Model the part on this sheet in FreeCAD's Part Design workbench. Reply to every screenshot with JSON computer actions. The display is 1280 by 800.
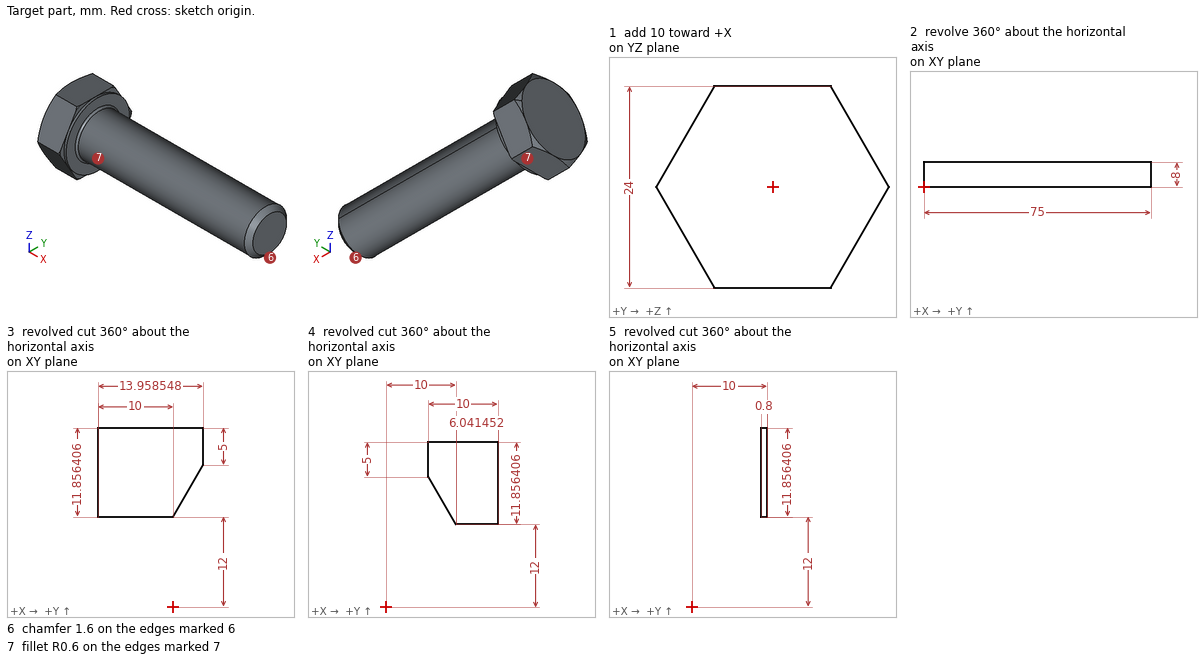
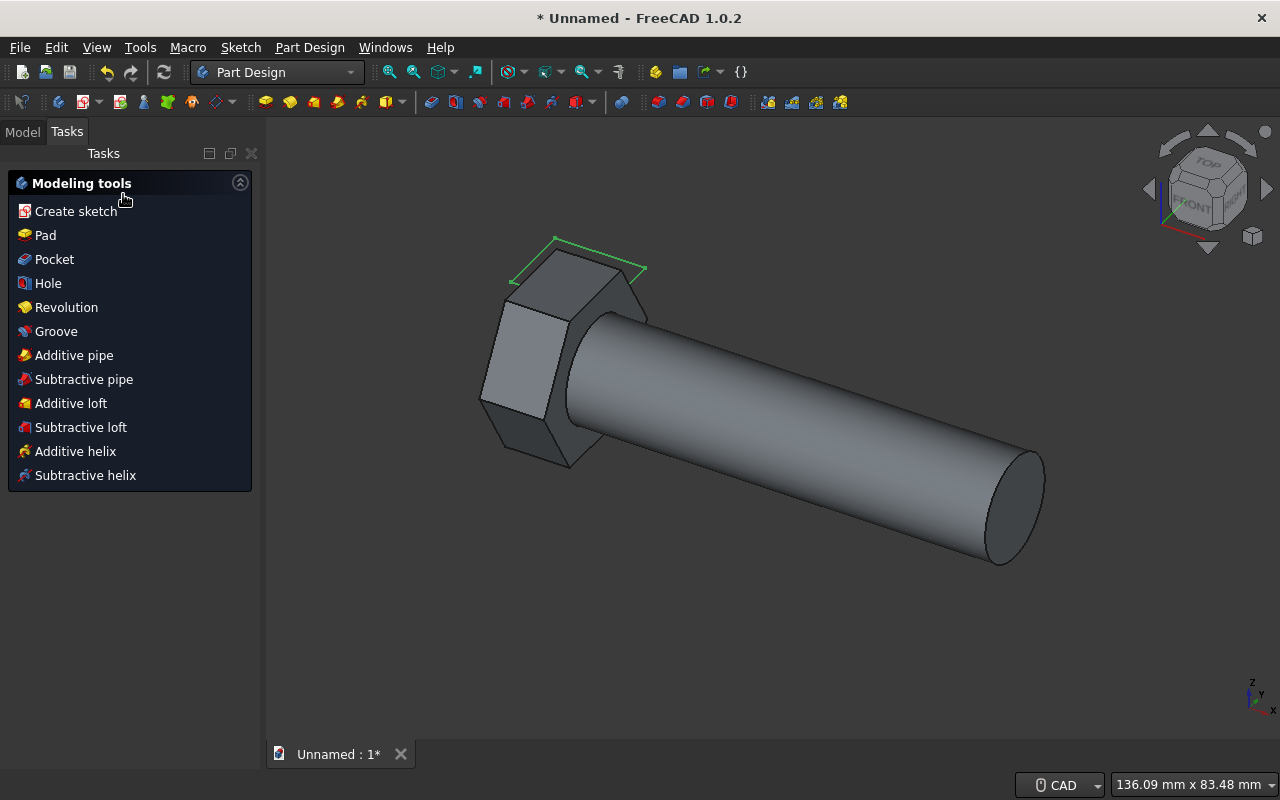
{"action": "left_click", "coordinate": [480, 102]}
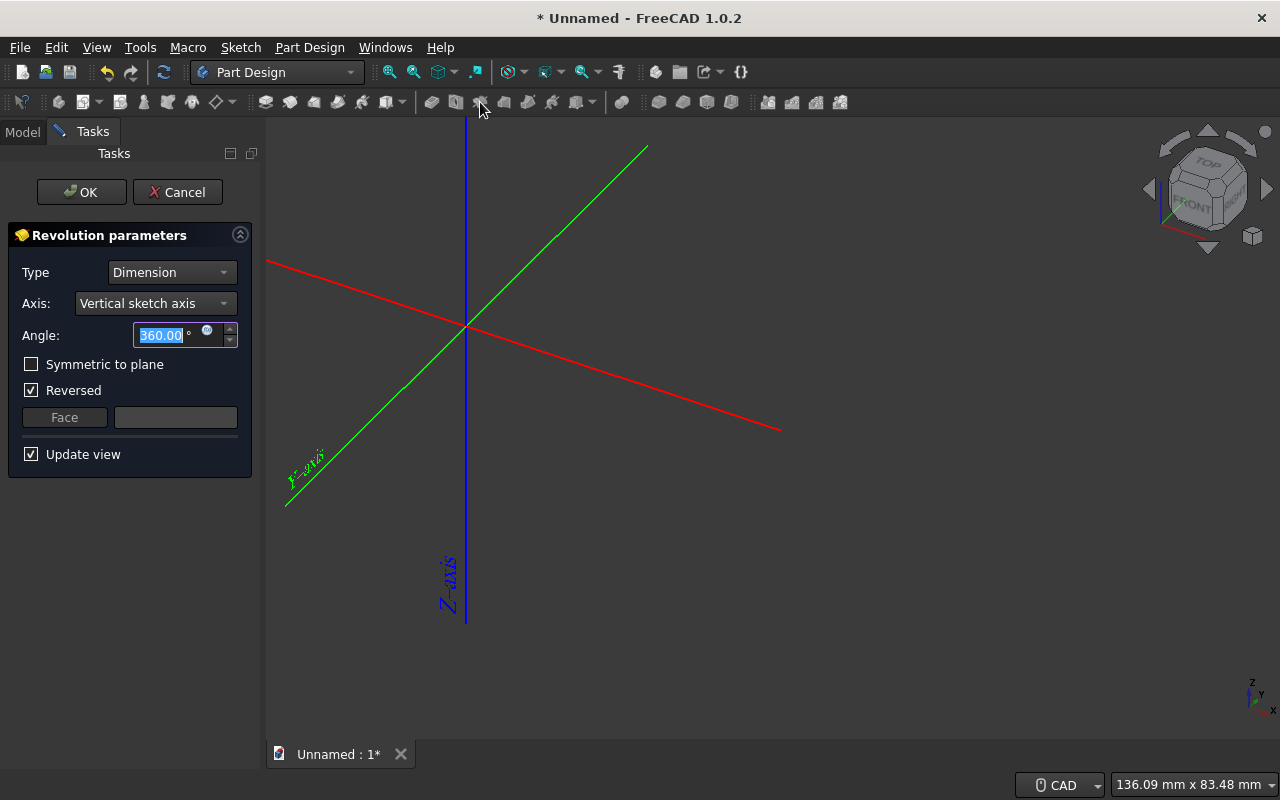
{"action": "left_click", "coordinate": [156, 304]}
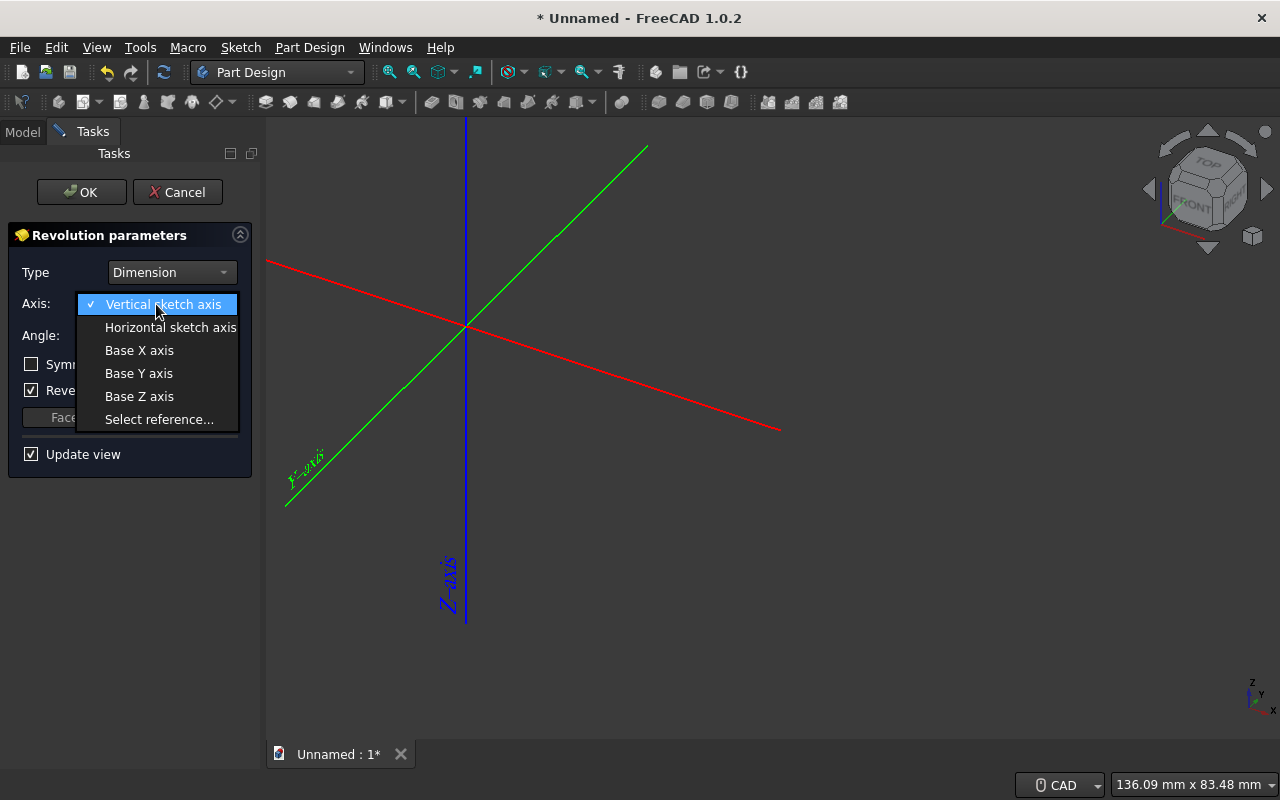
{"action": "left_click", "coordinate": [156, 328]}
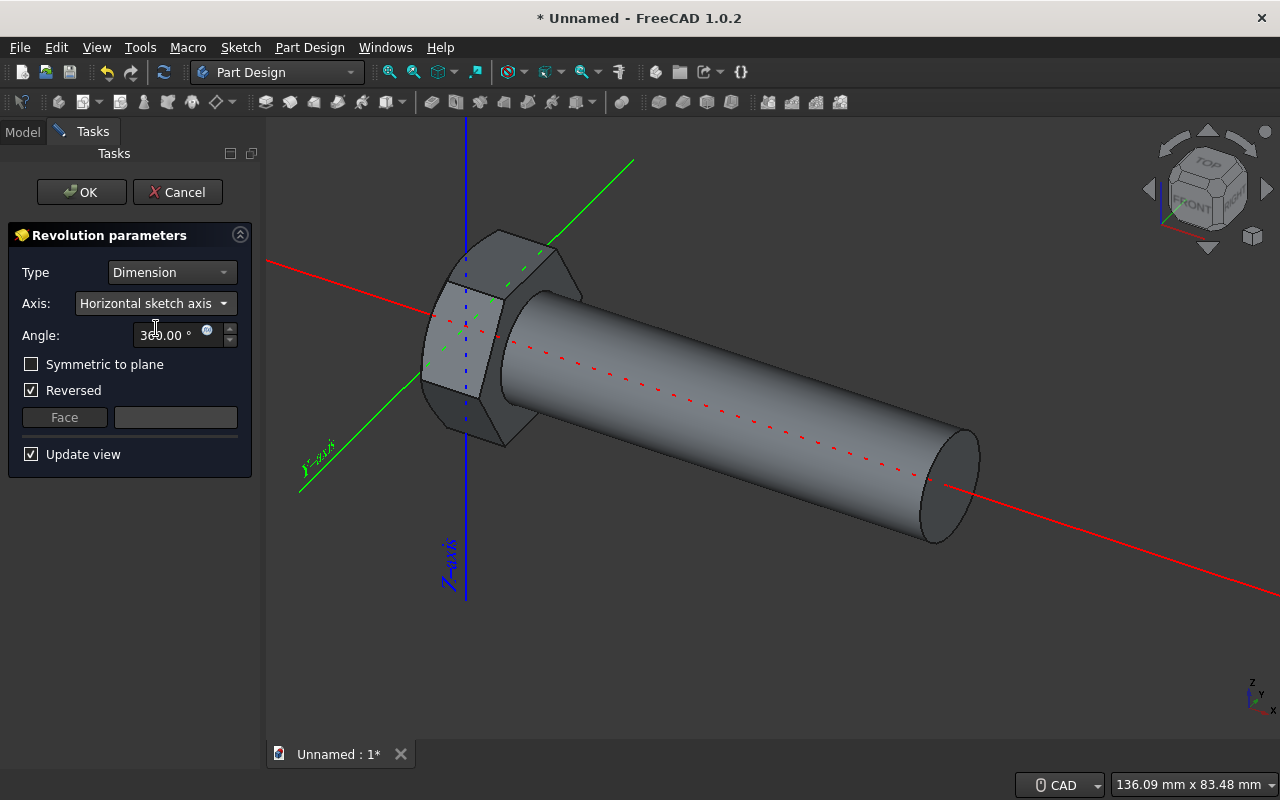
{"action": "left_click", "coordinate": [82, 192]}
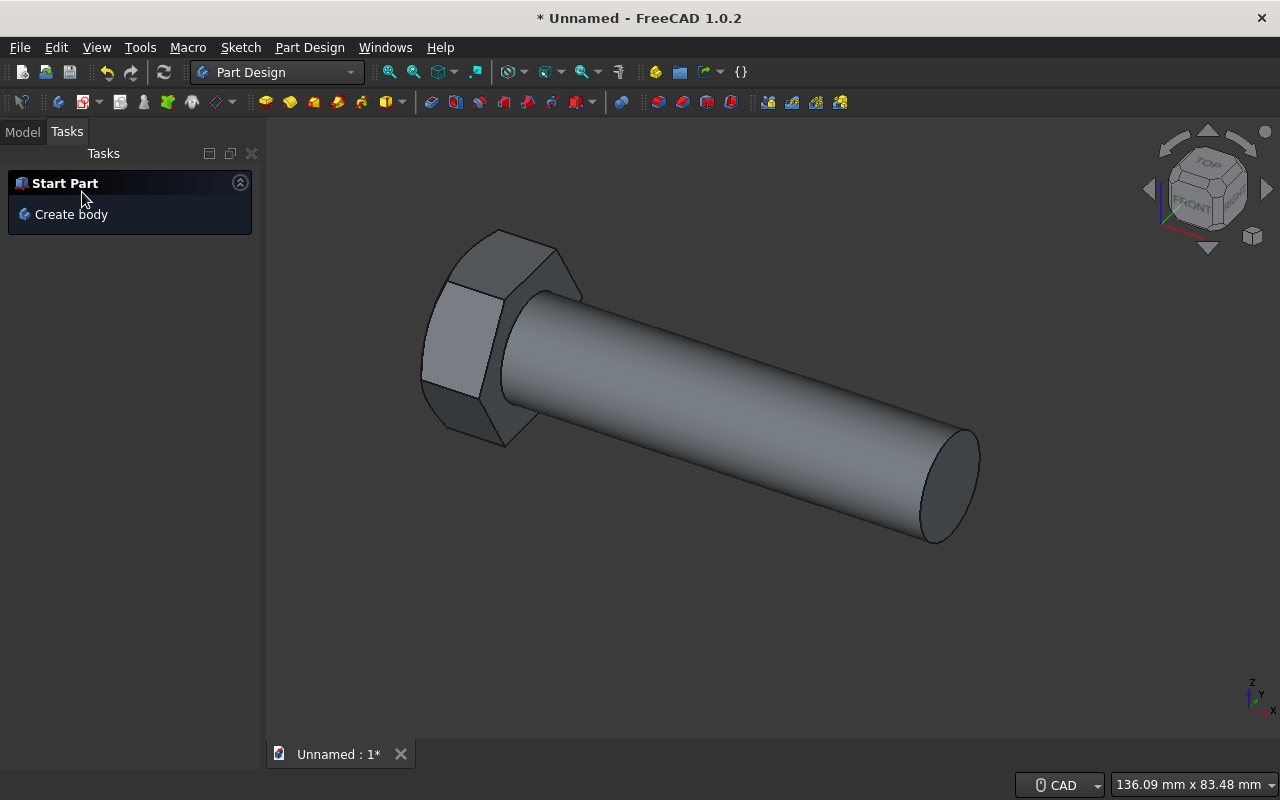
{"action": "left_click", "coordinate": [84, 102]}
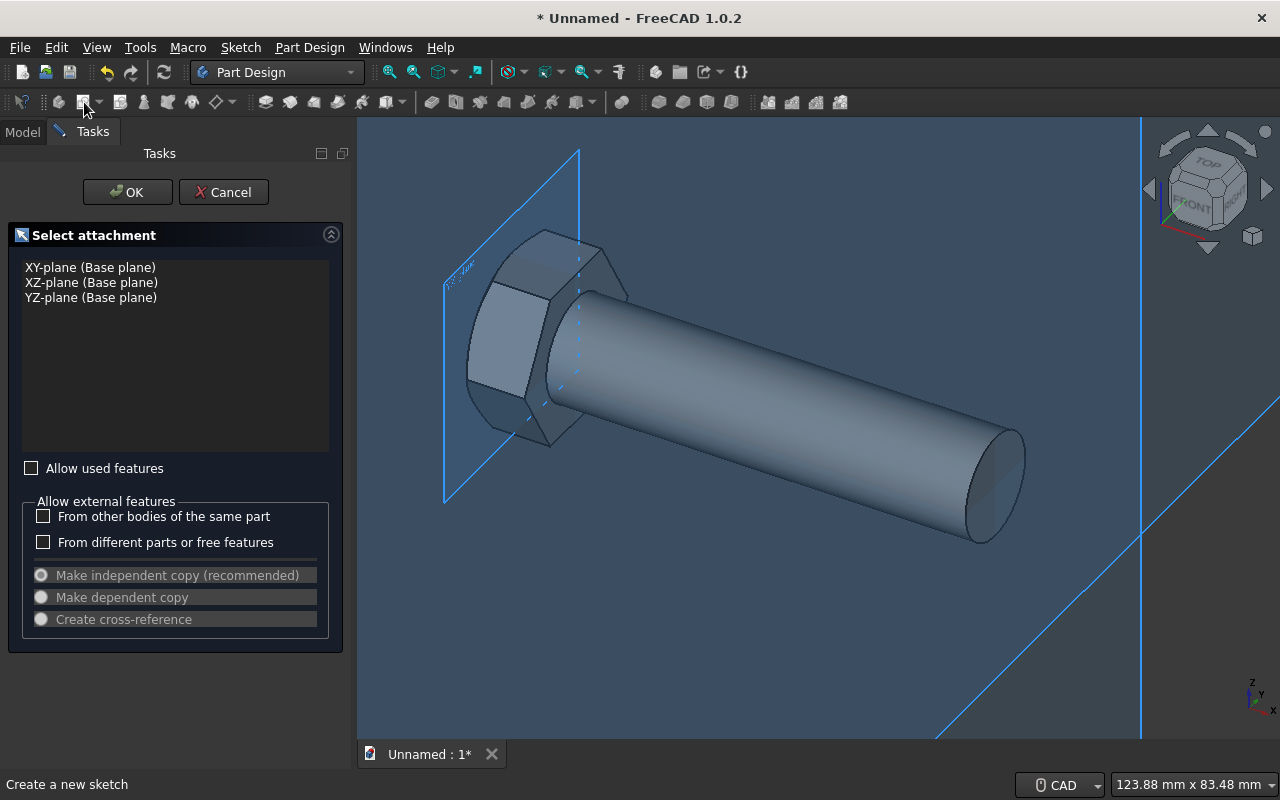
{"action": "left_click", "coordinate": [82, 268]}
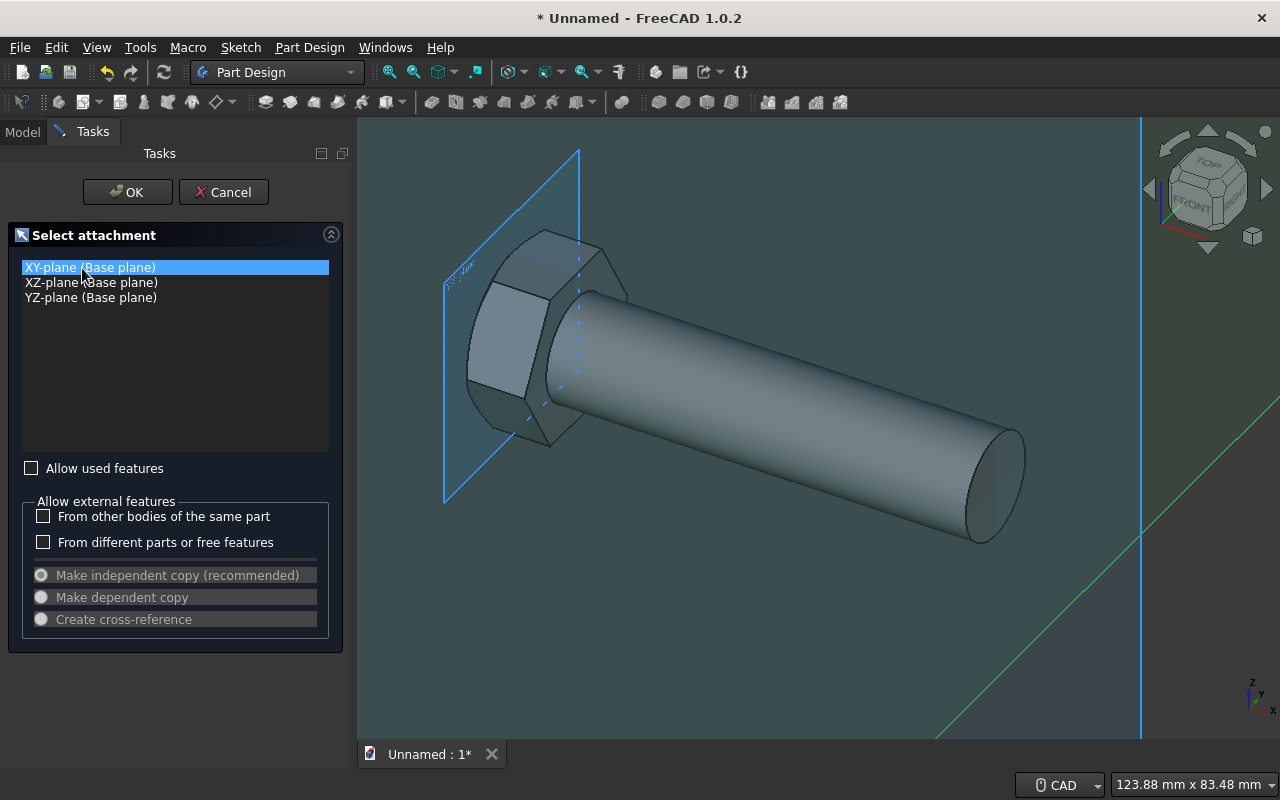
{"action": "left_click", "coordinate": [128, 192]}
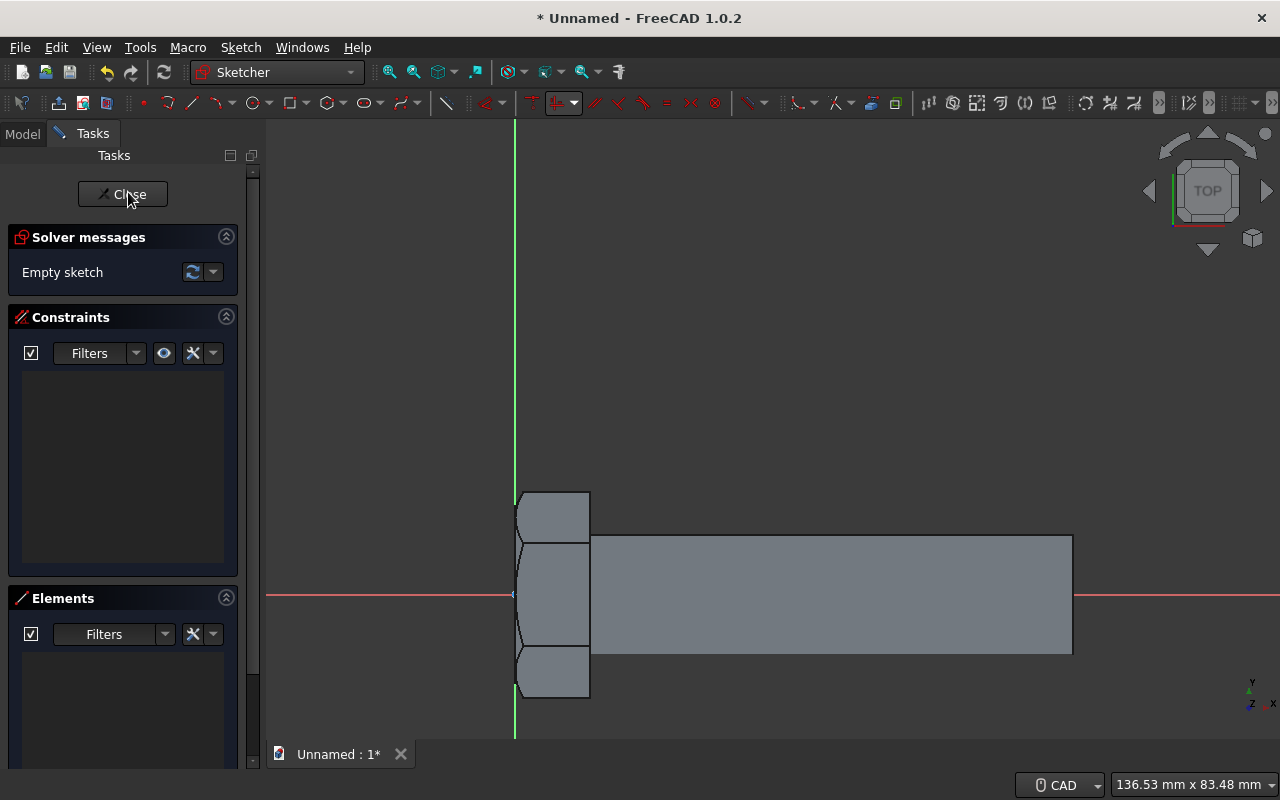
{"action": "left_click", "coordinate": [108, 104]}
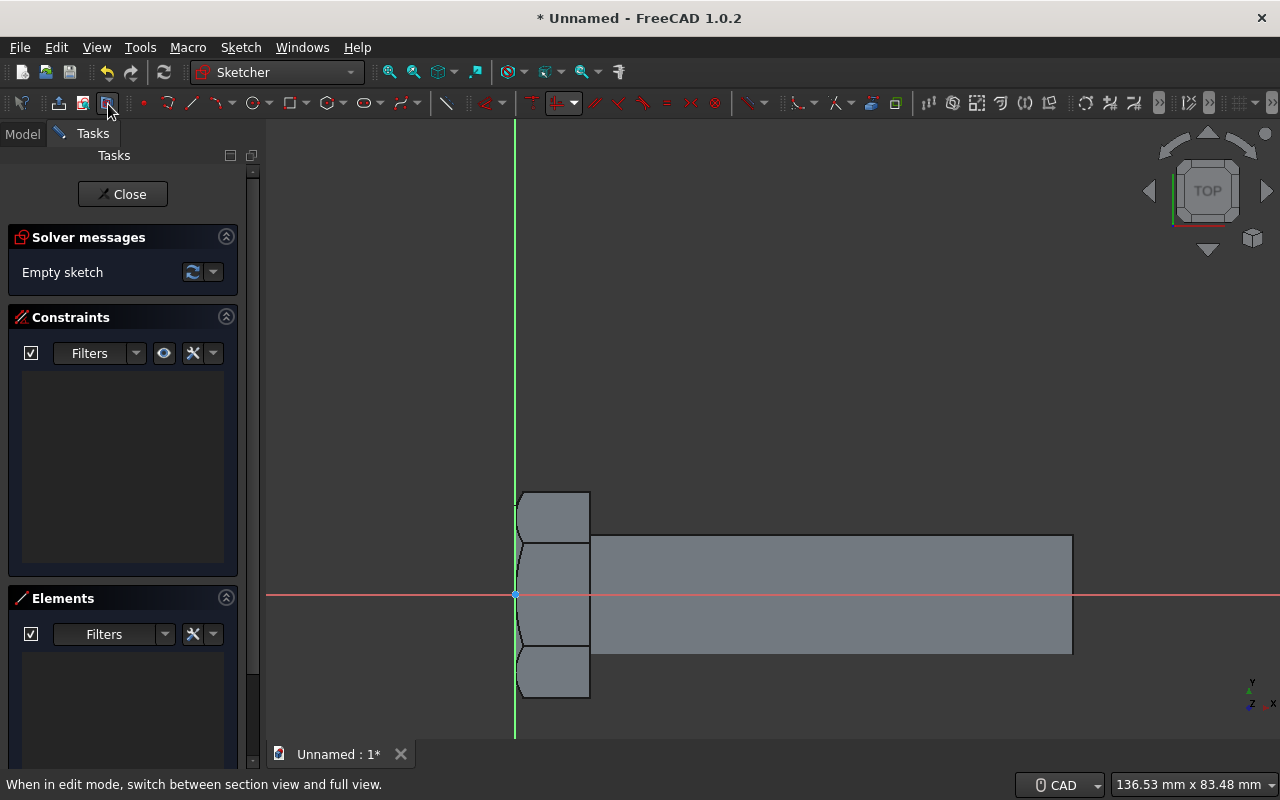
{"action": "scroll", "coordinate": [469, 569], "scroll_direction": "up", "scroll_amount": 4}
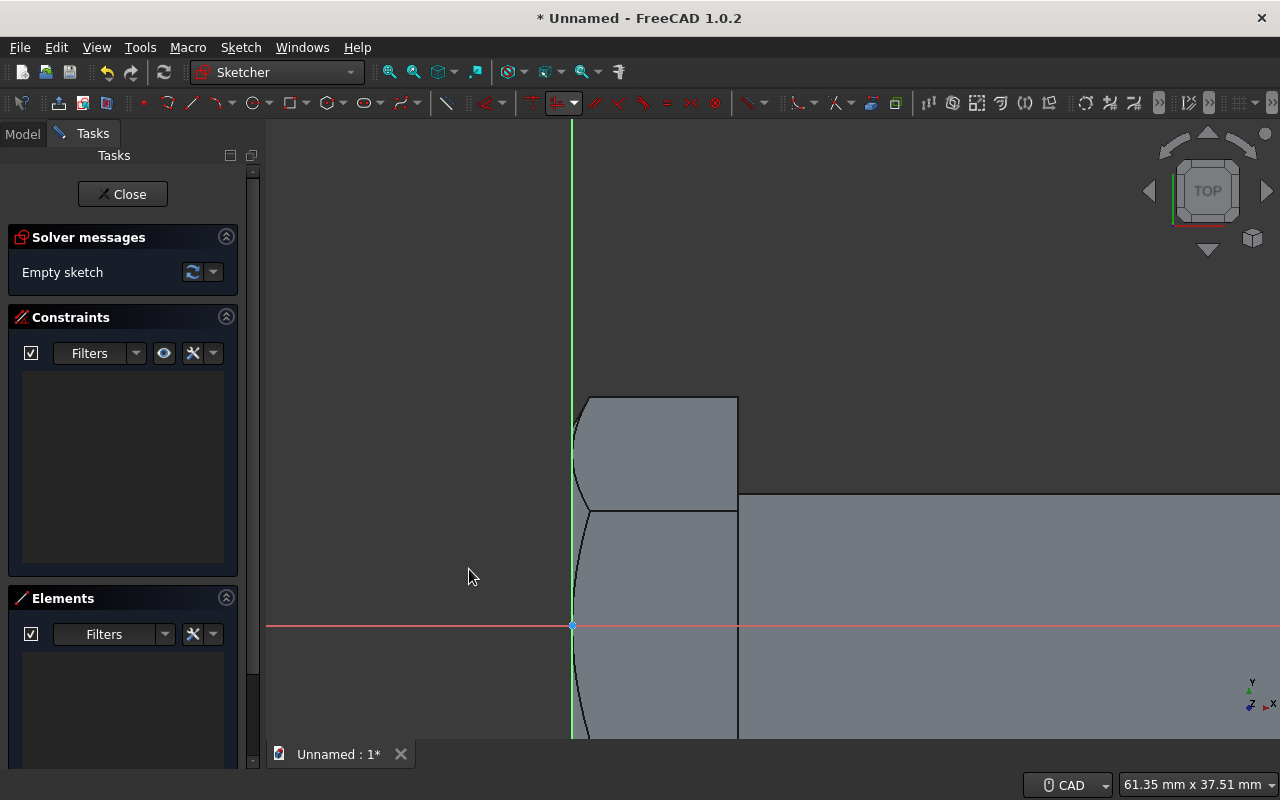
{"action": "left_click", "coordinate": [168, 104]}